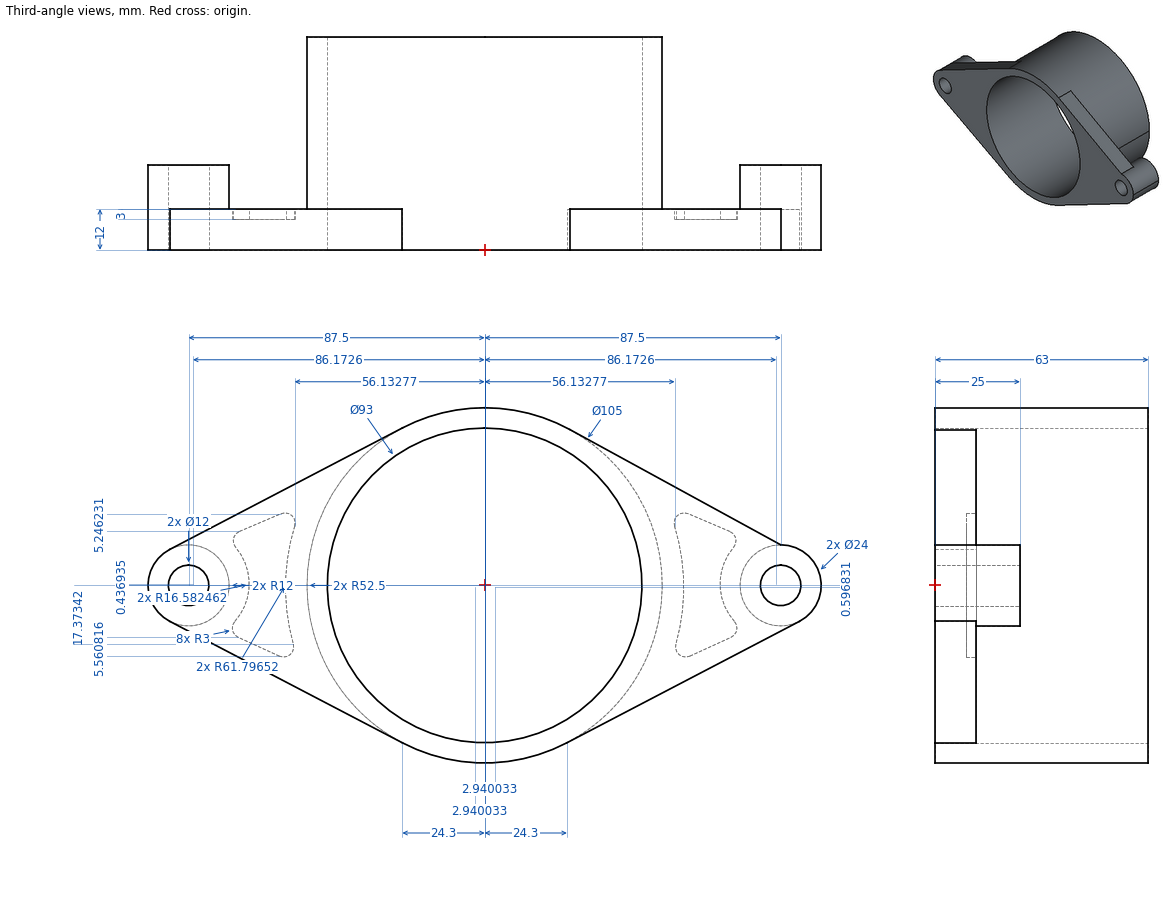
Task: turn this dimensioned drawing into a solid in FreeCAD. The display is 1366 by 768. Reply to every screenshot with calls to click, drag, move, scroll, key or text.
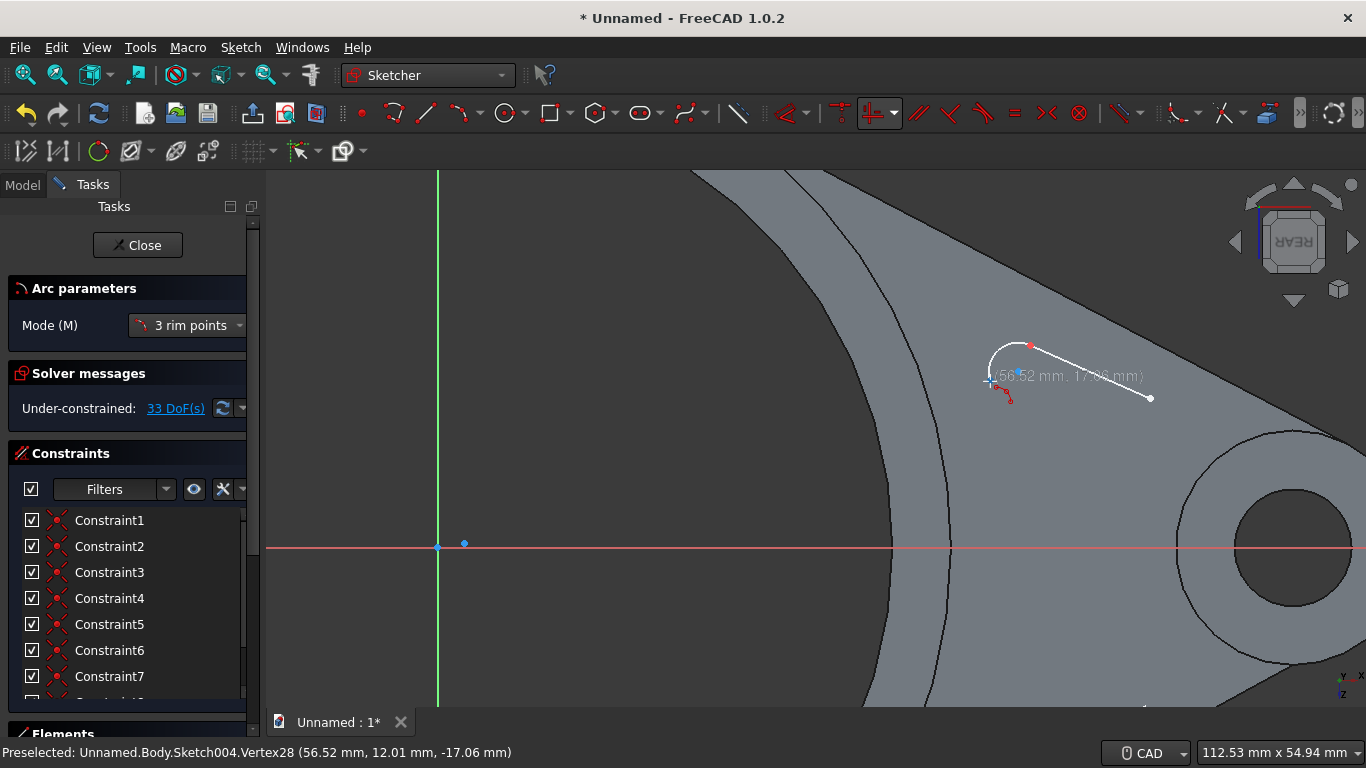
scroll(1000, 348, down, 4)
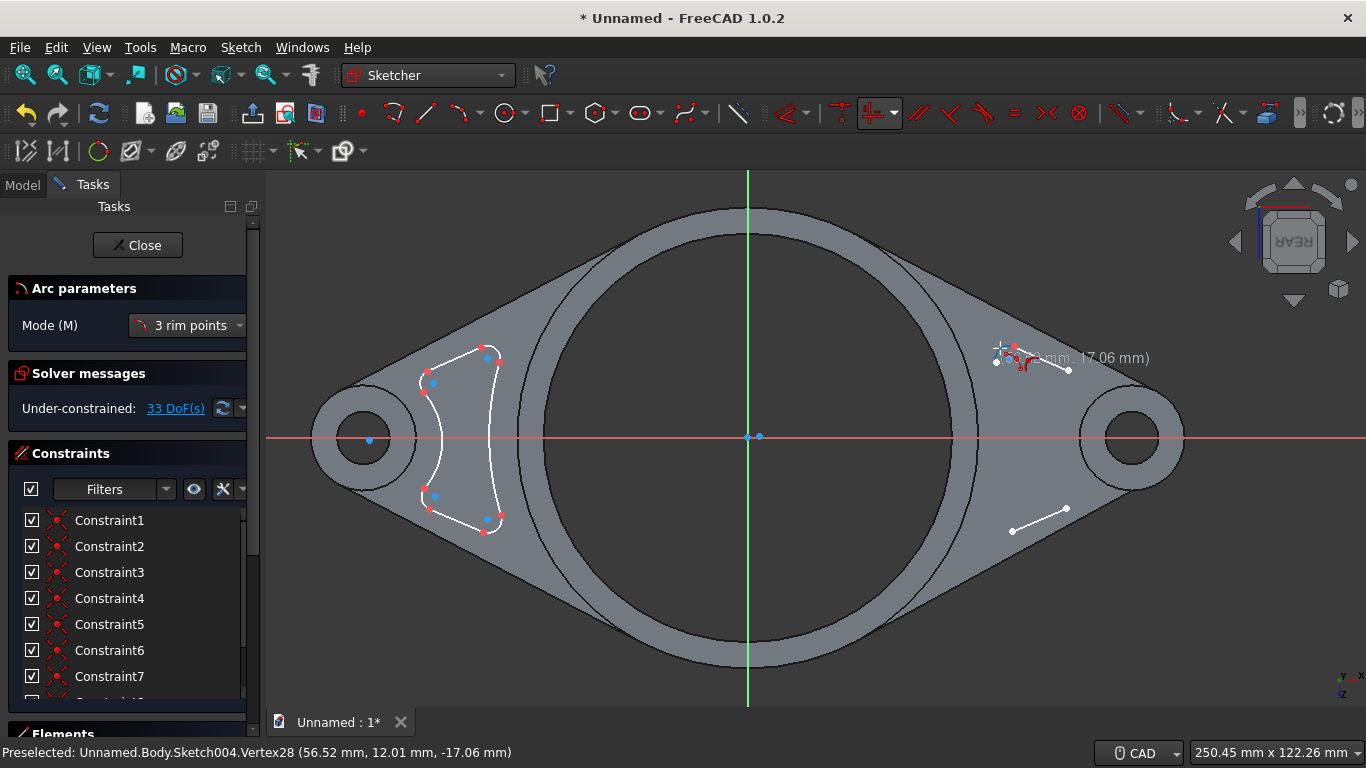
click(994, 515)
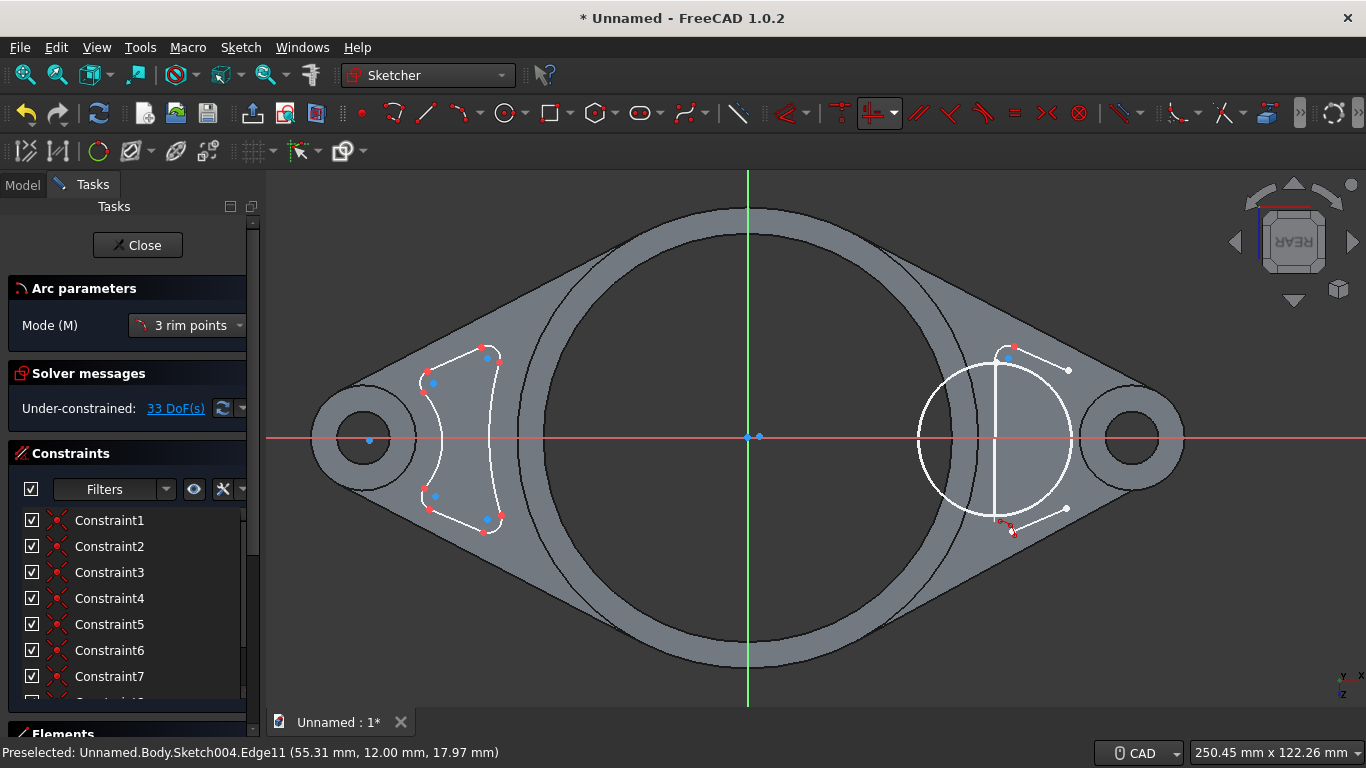
scroll(1006, 423, up, 3)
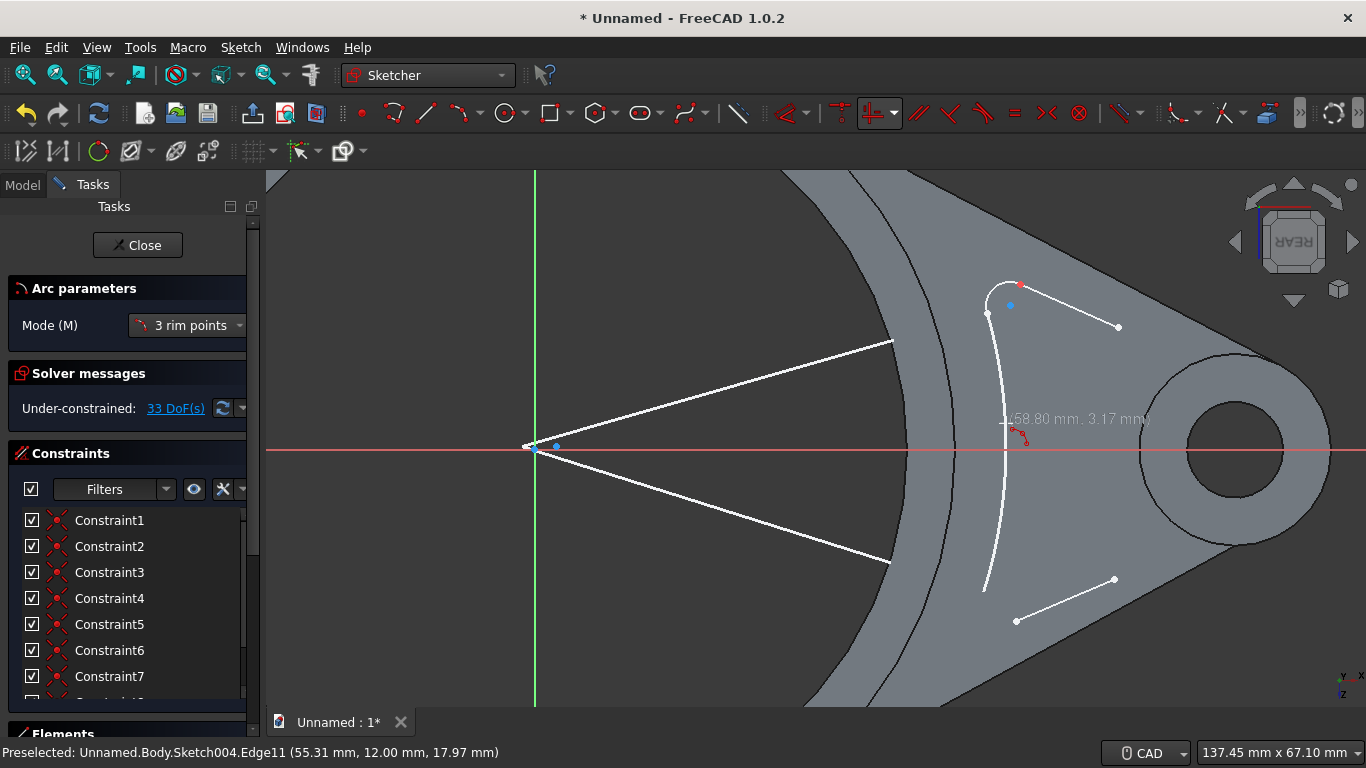
click(1005, 422)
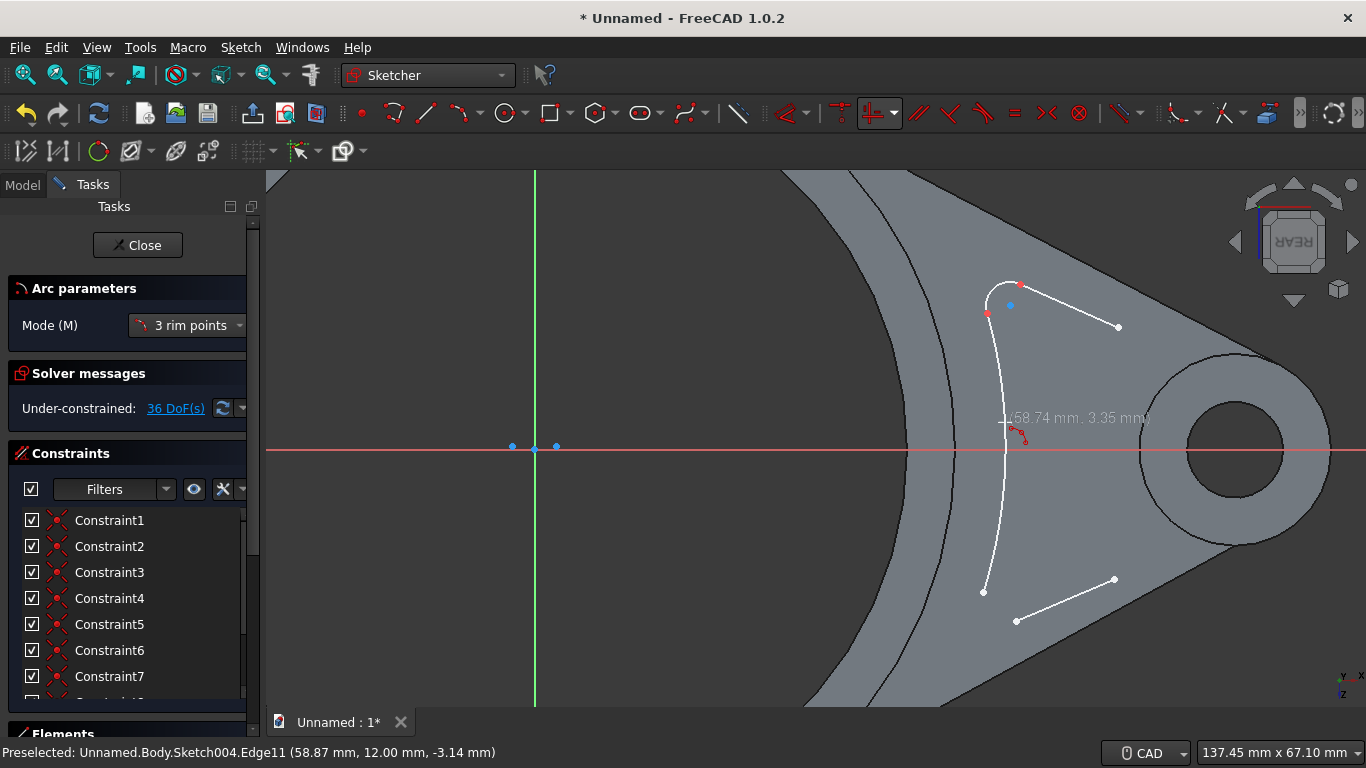
click(984, 592)
click(1016, 621)
click(991, 615)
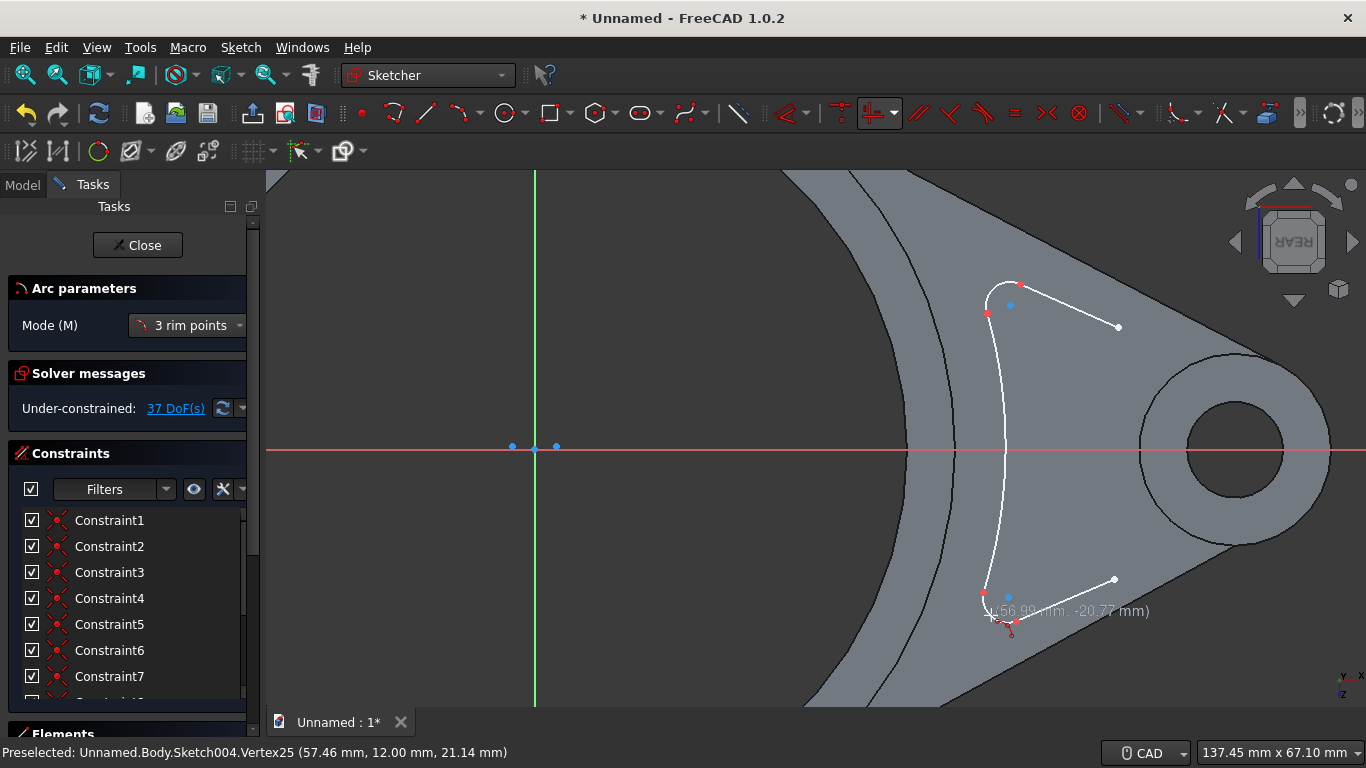
click(1115, 579)
click(1124, 540)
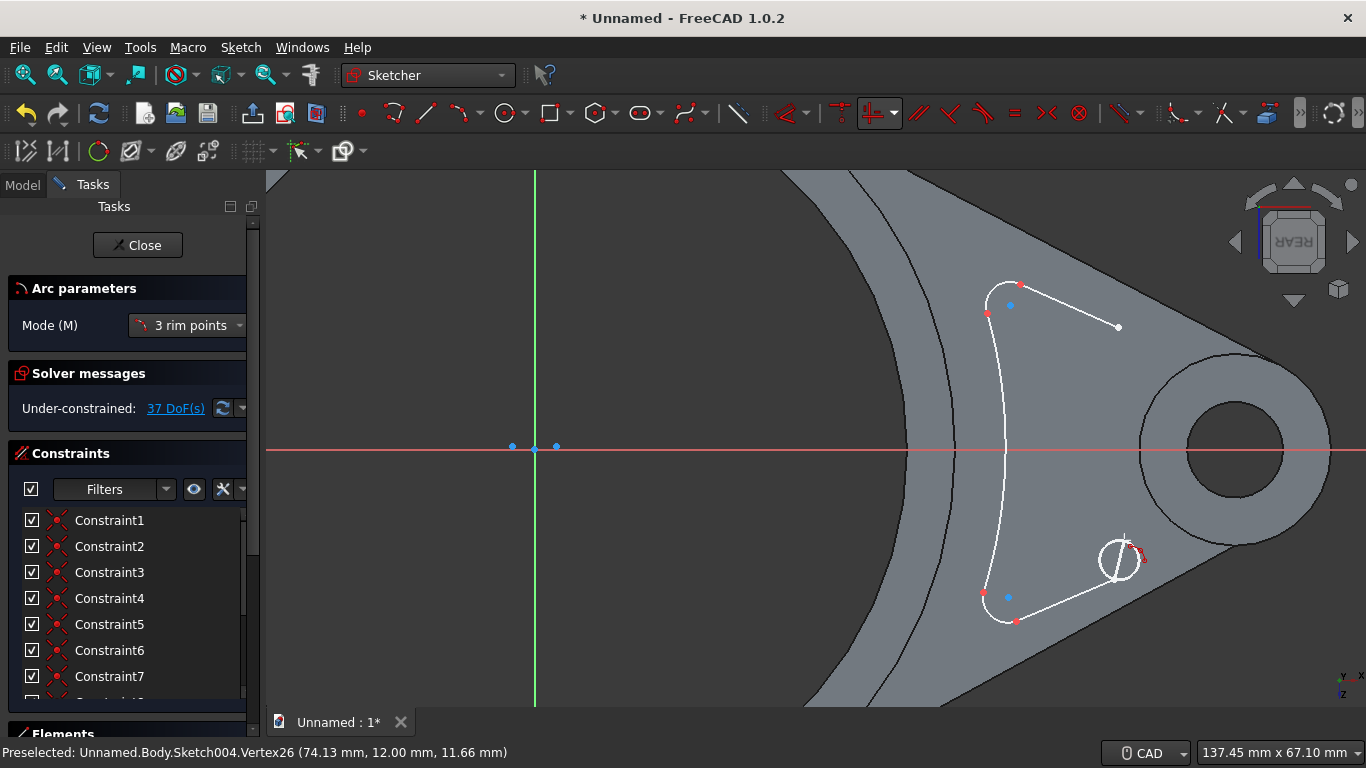
scroll(1129, 561, up, 3)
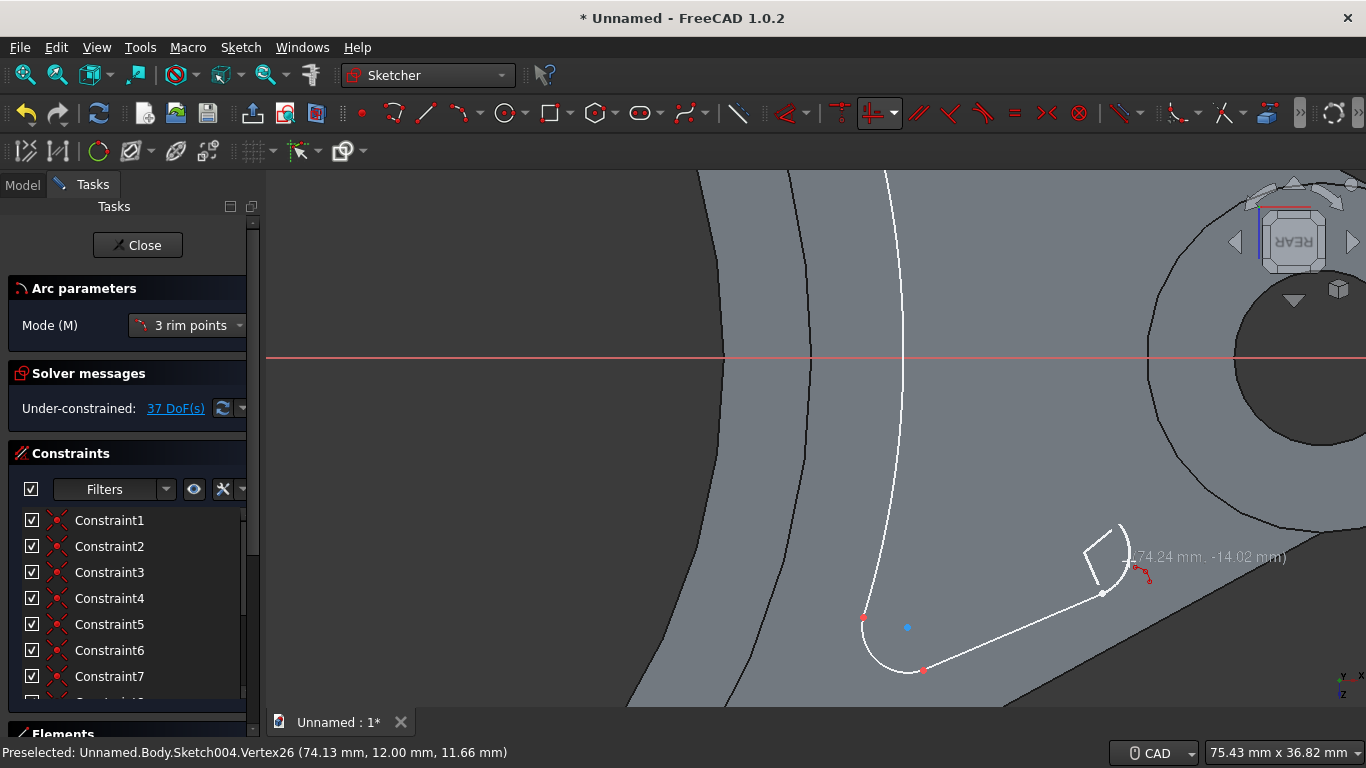
click(1128, 560)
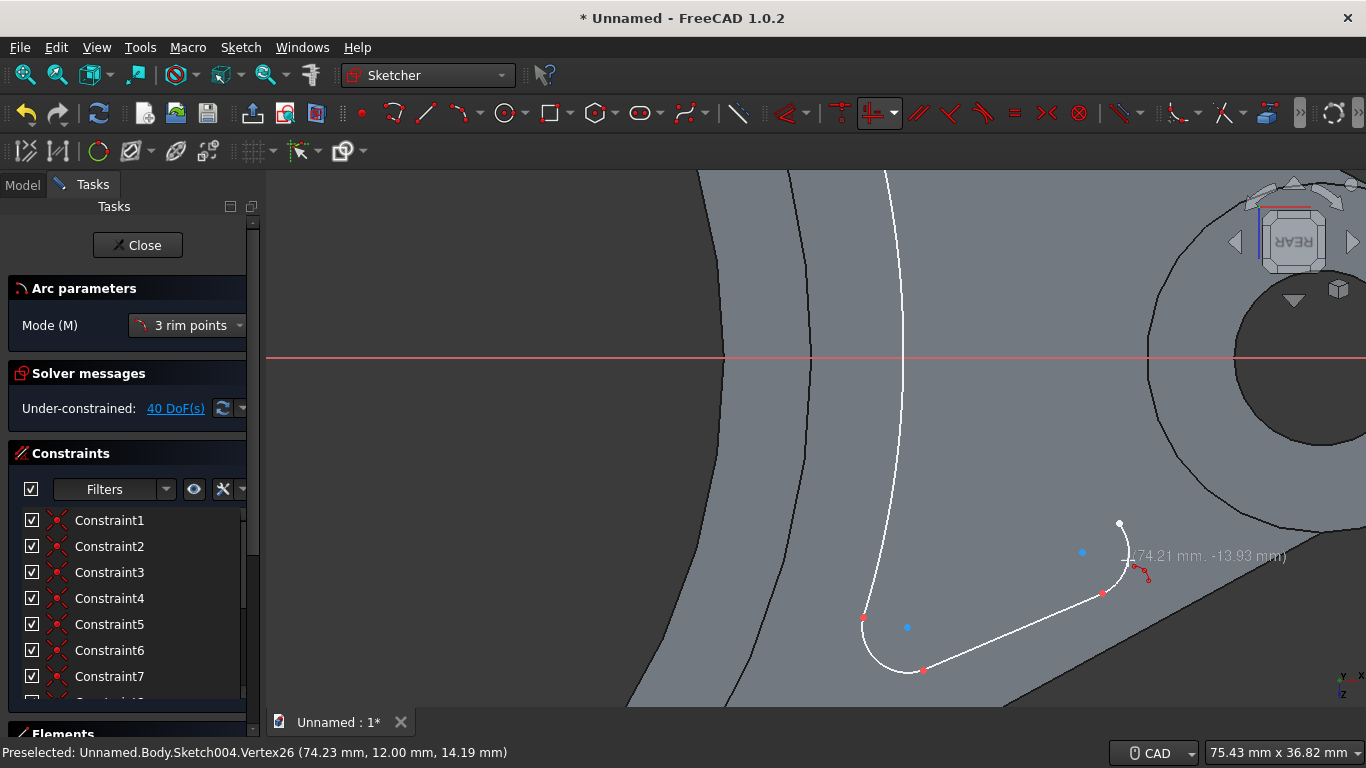
click(1119, 524)
click(1122, 203)
click(1071, 293)